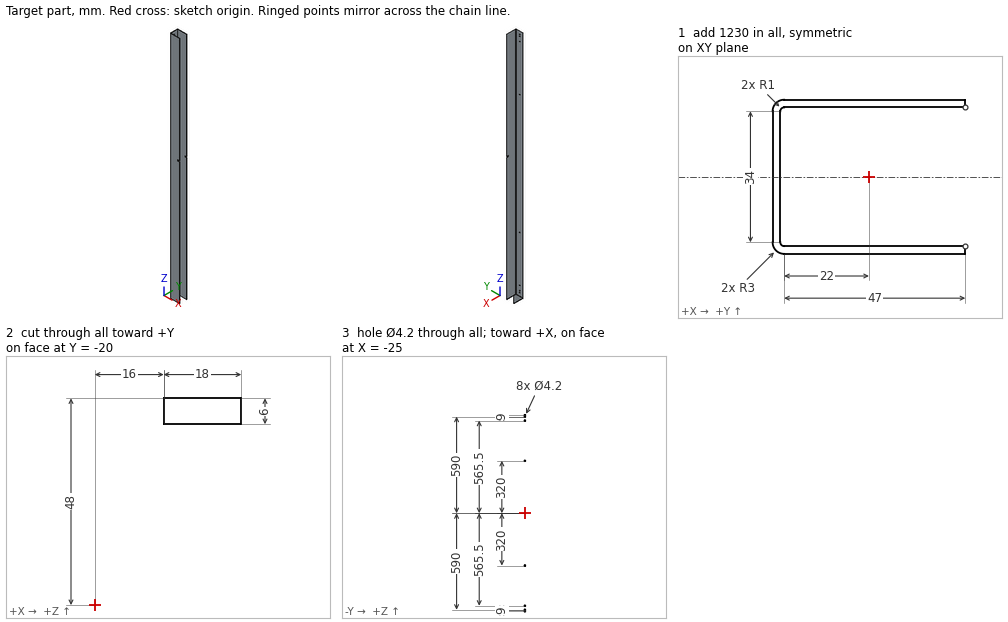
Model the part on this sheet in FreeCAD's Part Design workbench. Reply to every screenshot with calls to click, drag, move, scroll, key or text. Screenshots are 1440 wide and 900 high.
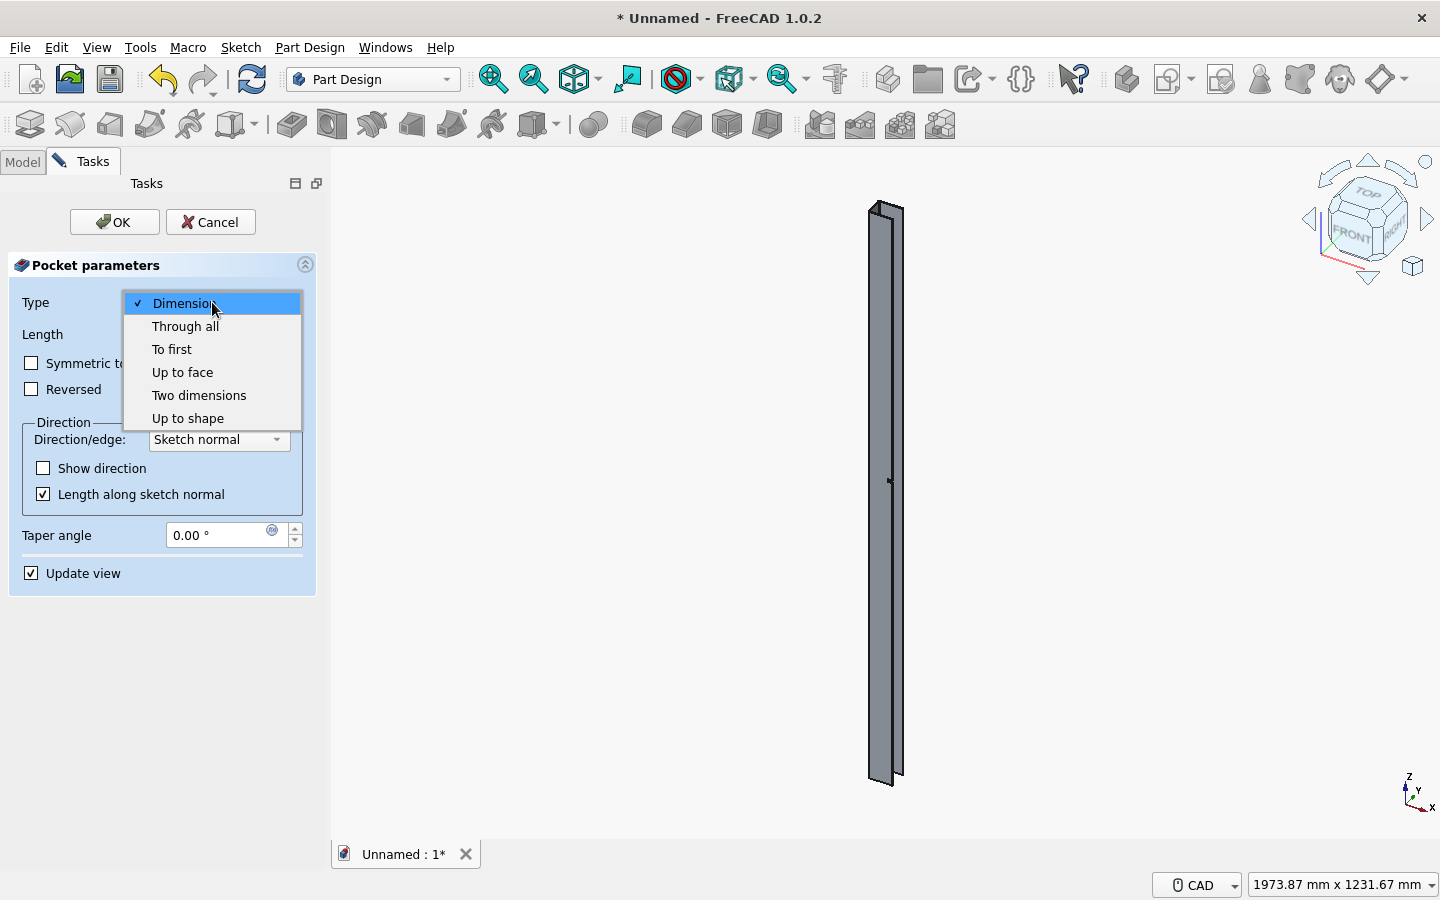
click(212, 326)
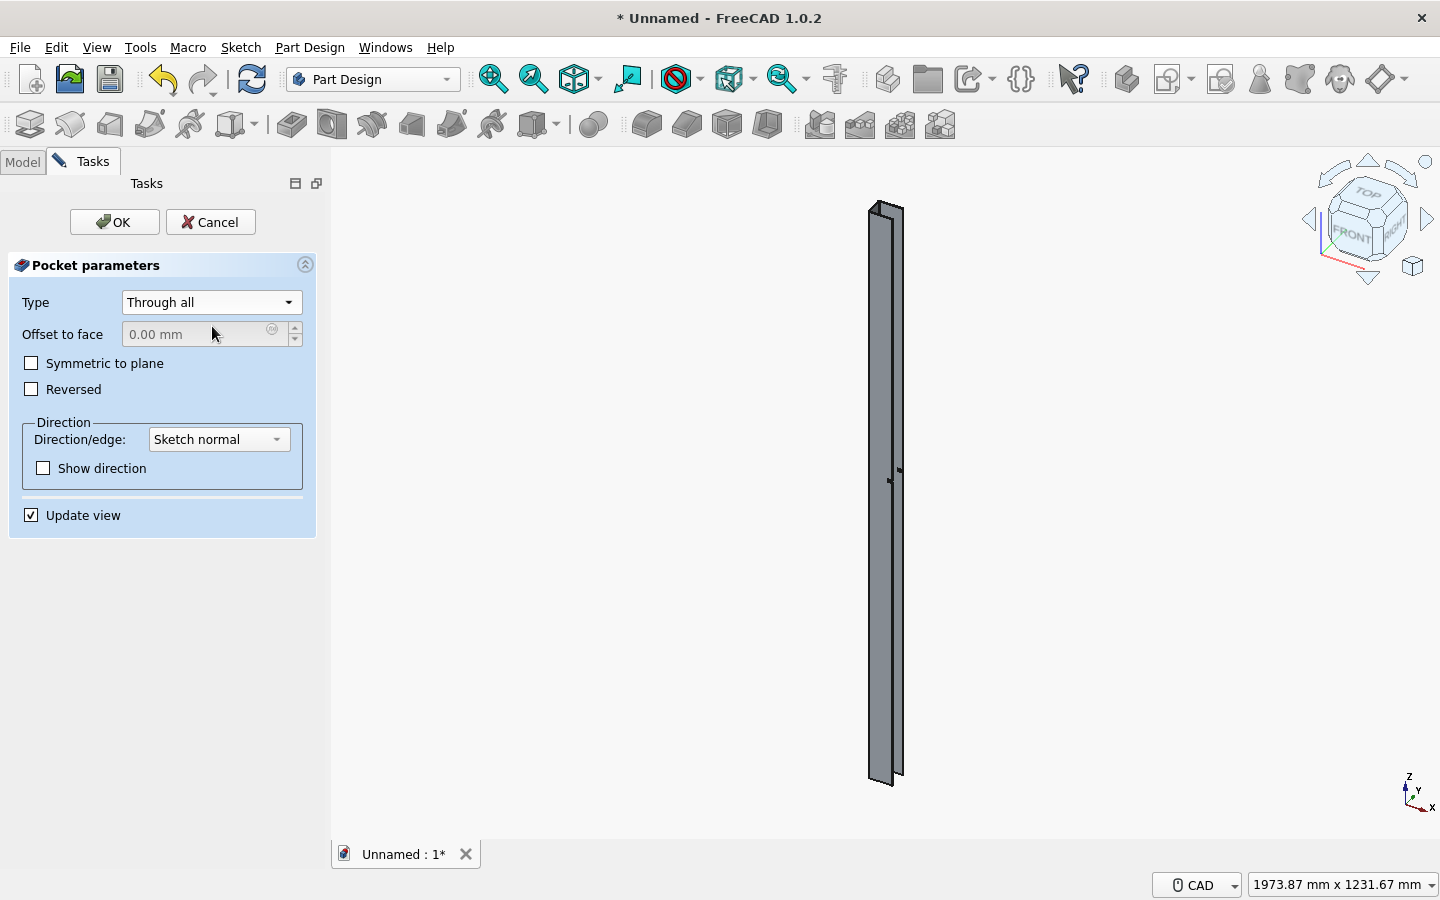
click(115, 222)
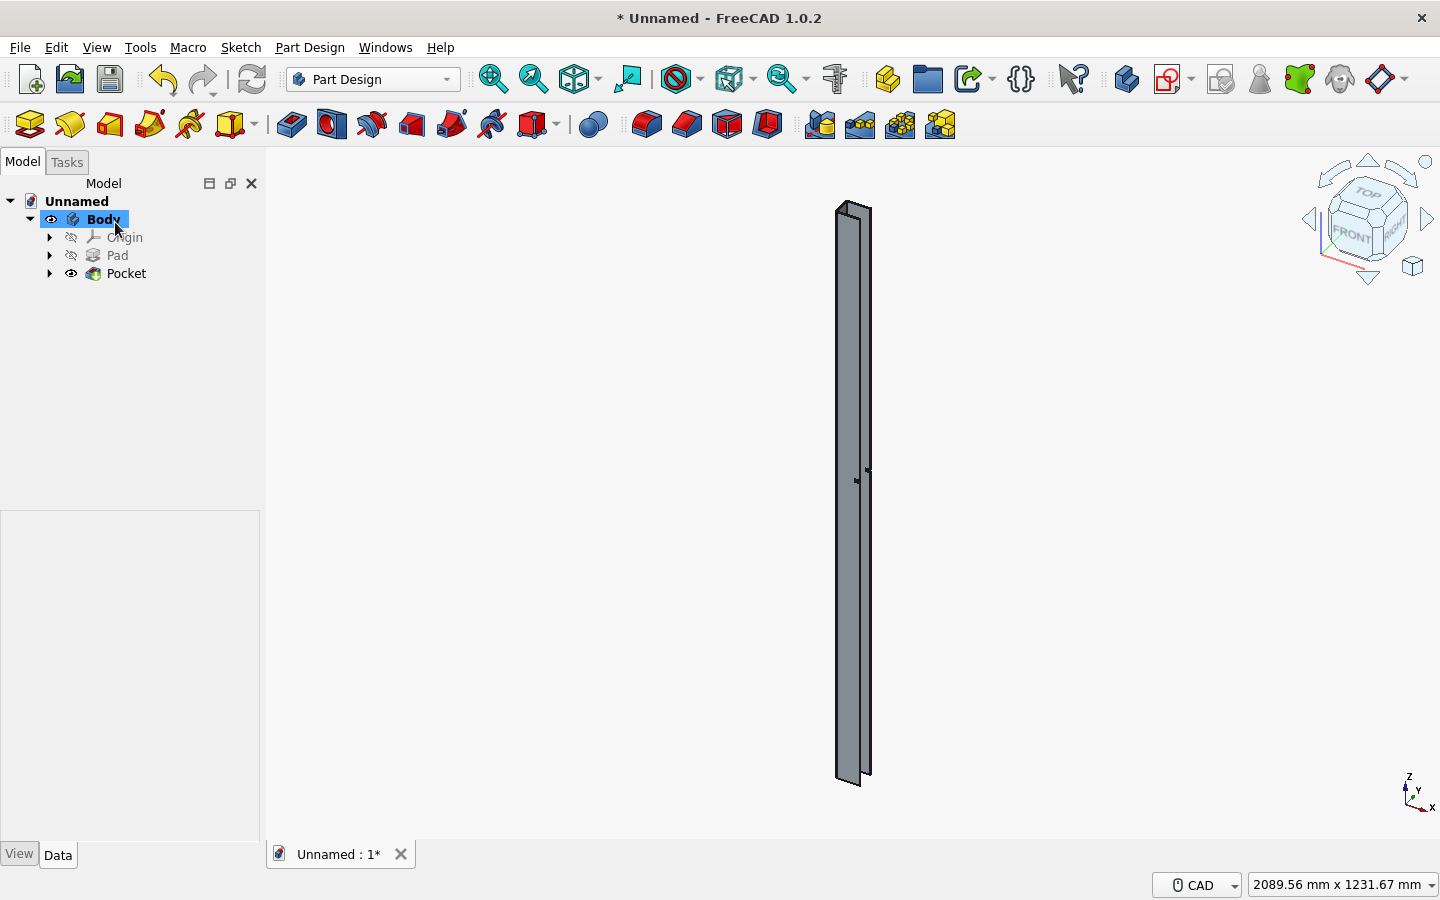
key(6)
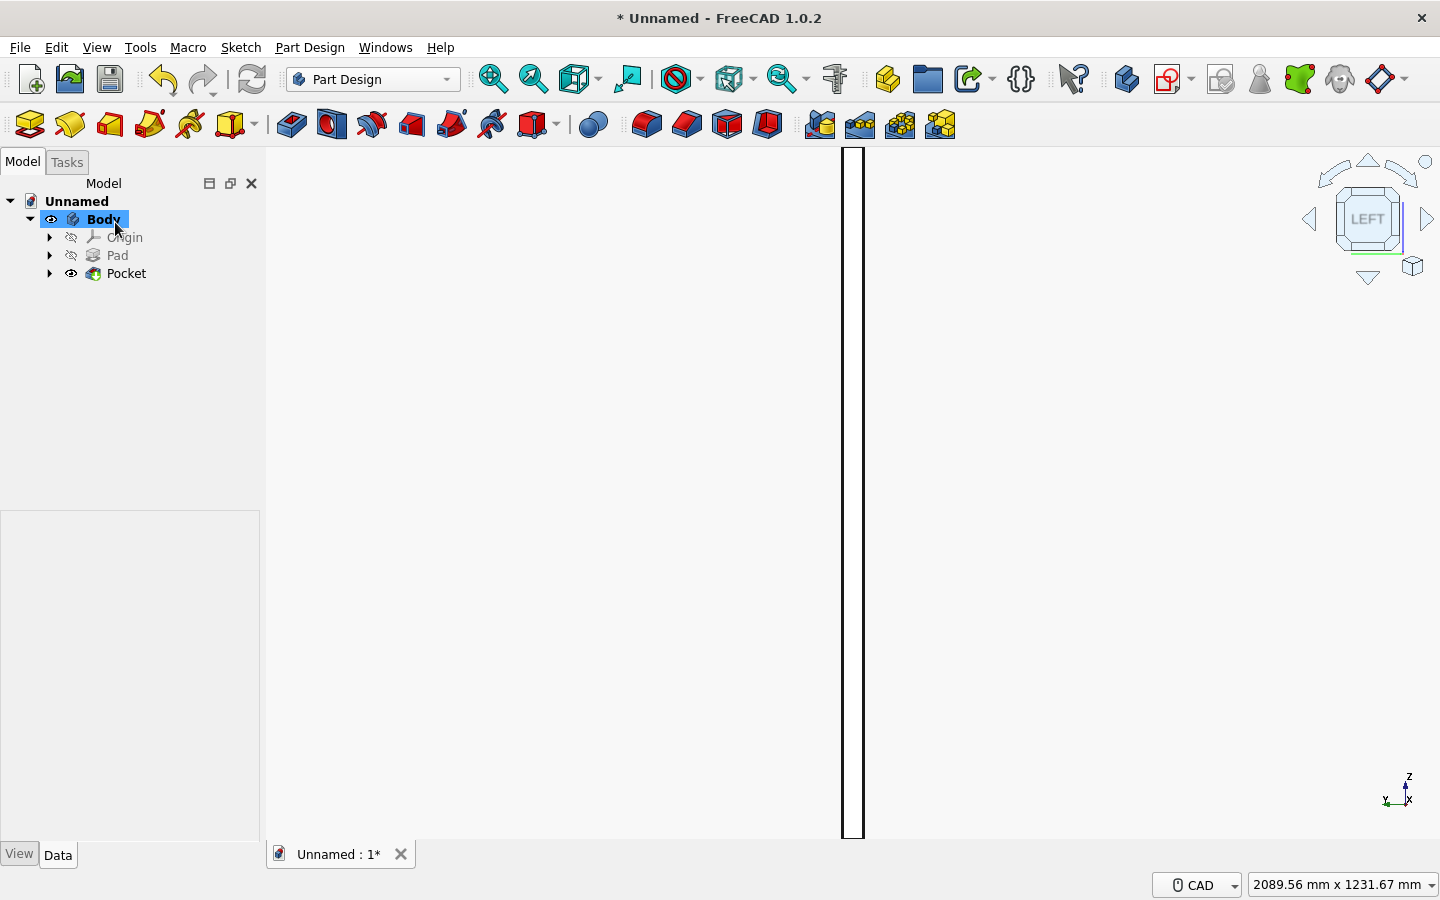
key(v)
key(f)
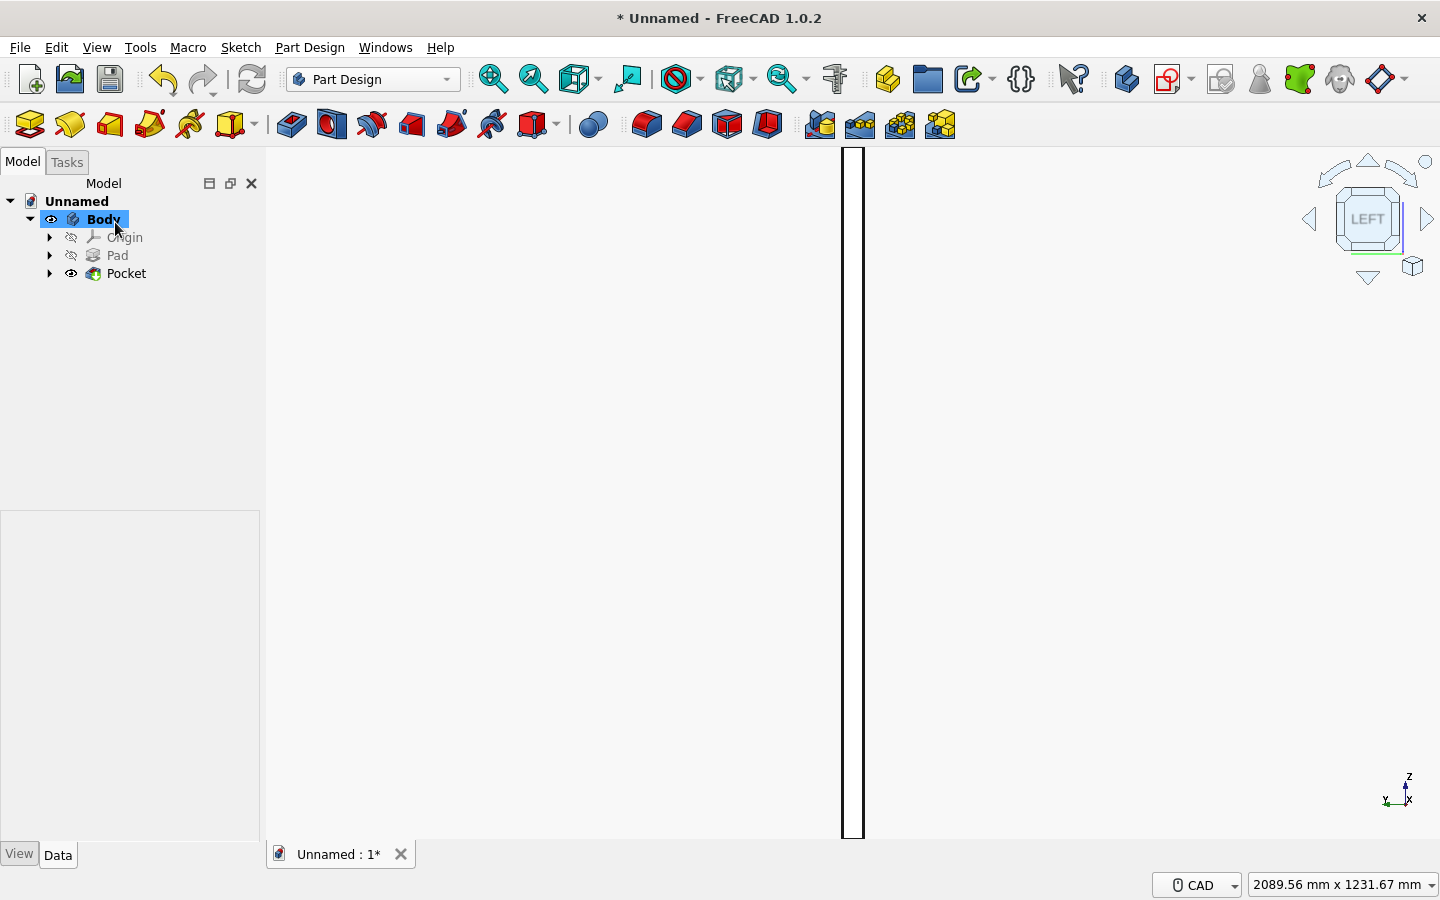
click(853, 196)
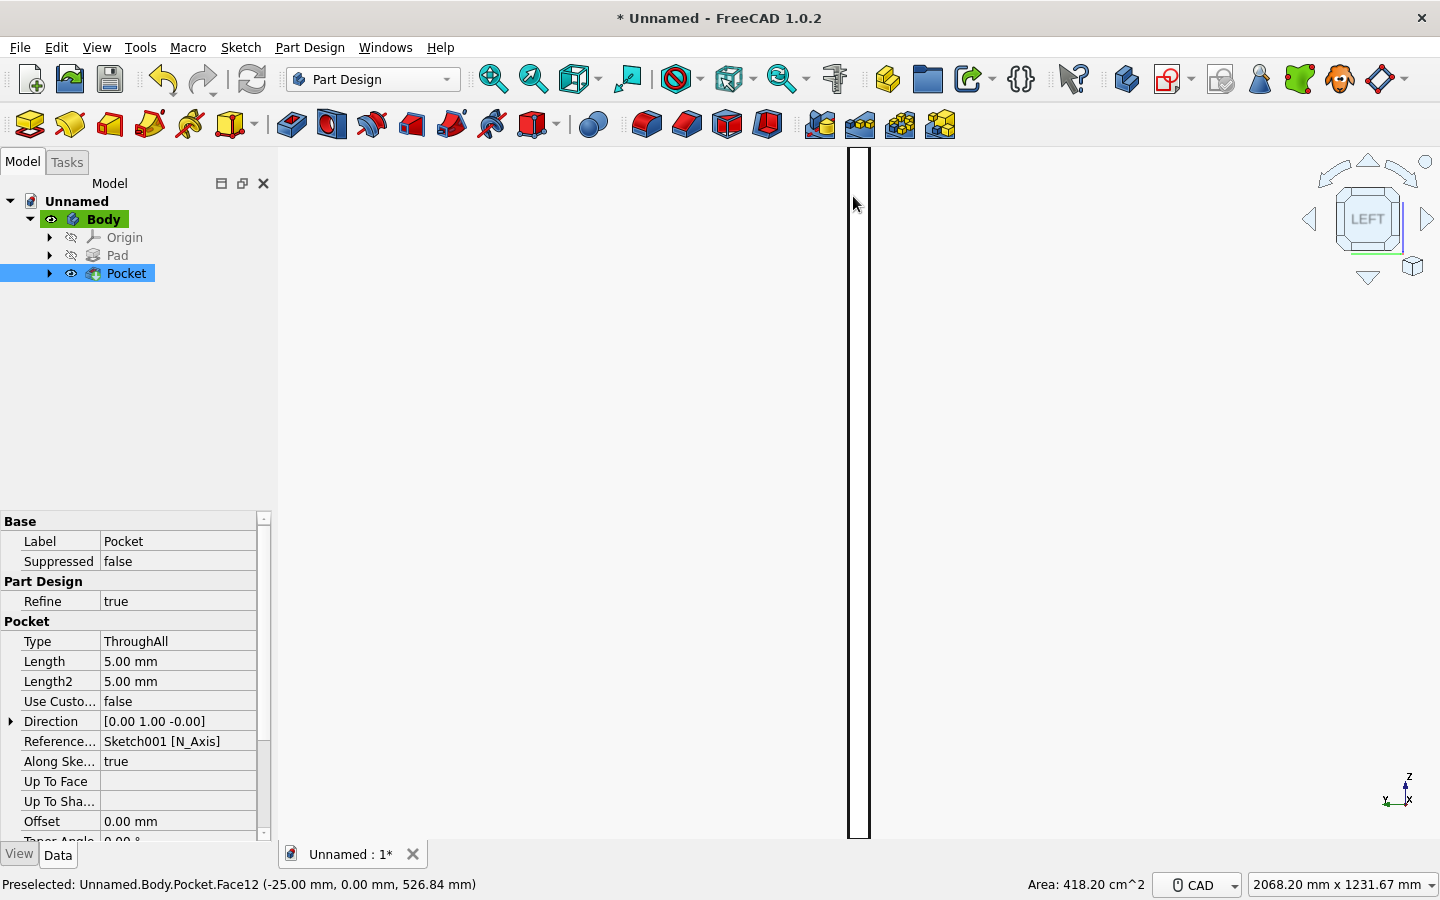
click(1168, 80)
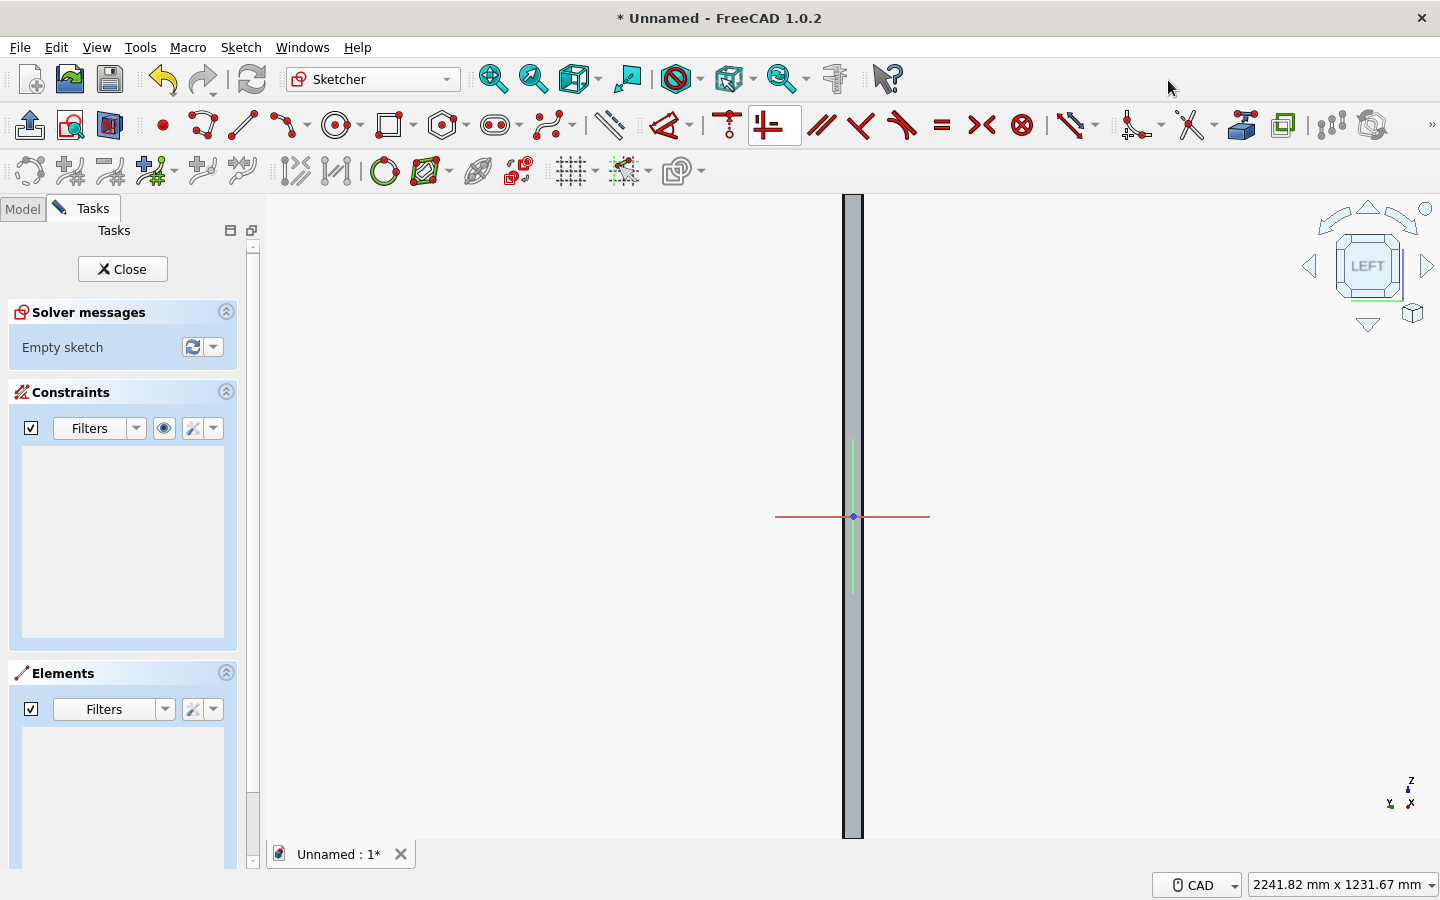
scroll(645, 516, down, 2)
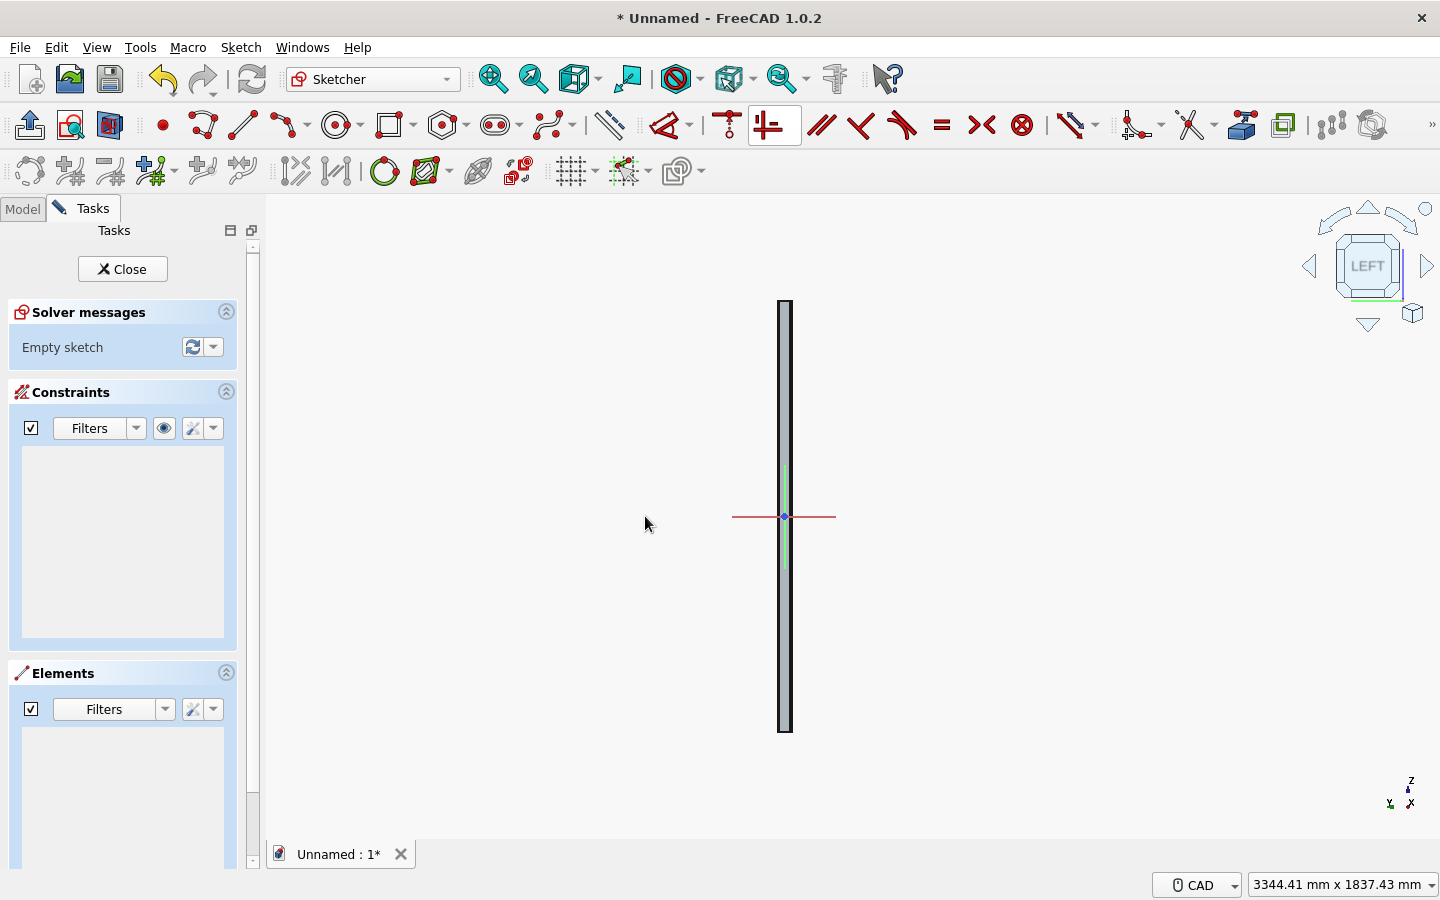
click(336, 126)